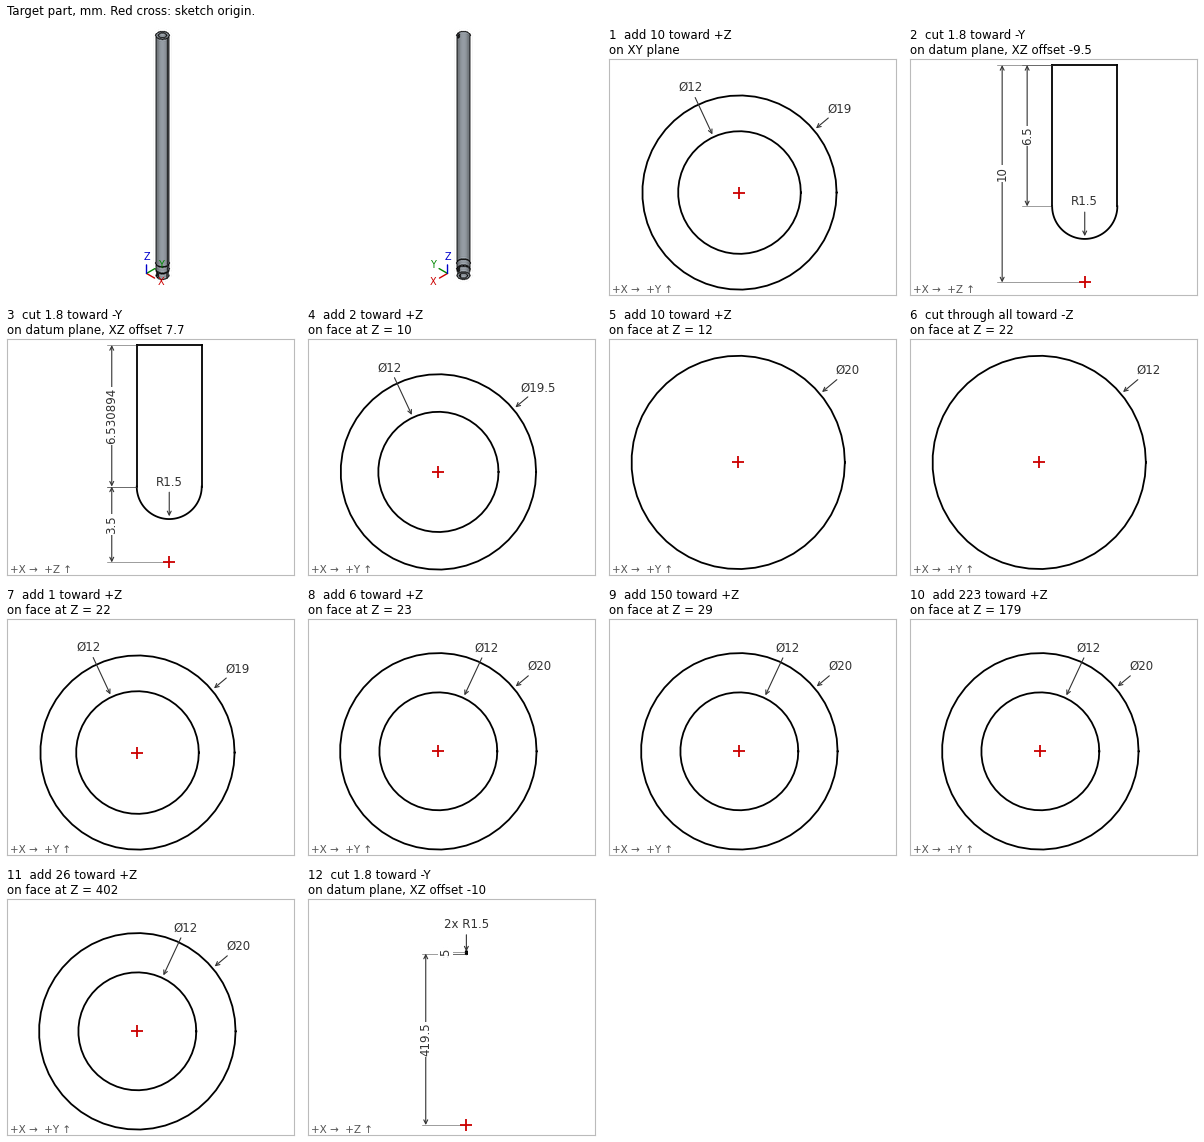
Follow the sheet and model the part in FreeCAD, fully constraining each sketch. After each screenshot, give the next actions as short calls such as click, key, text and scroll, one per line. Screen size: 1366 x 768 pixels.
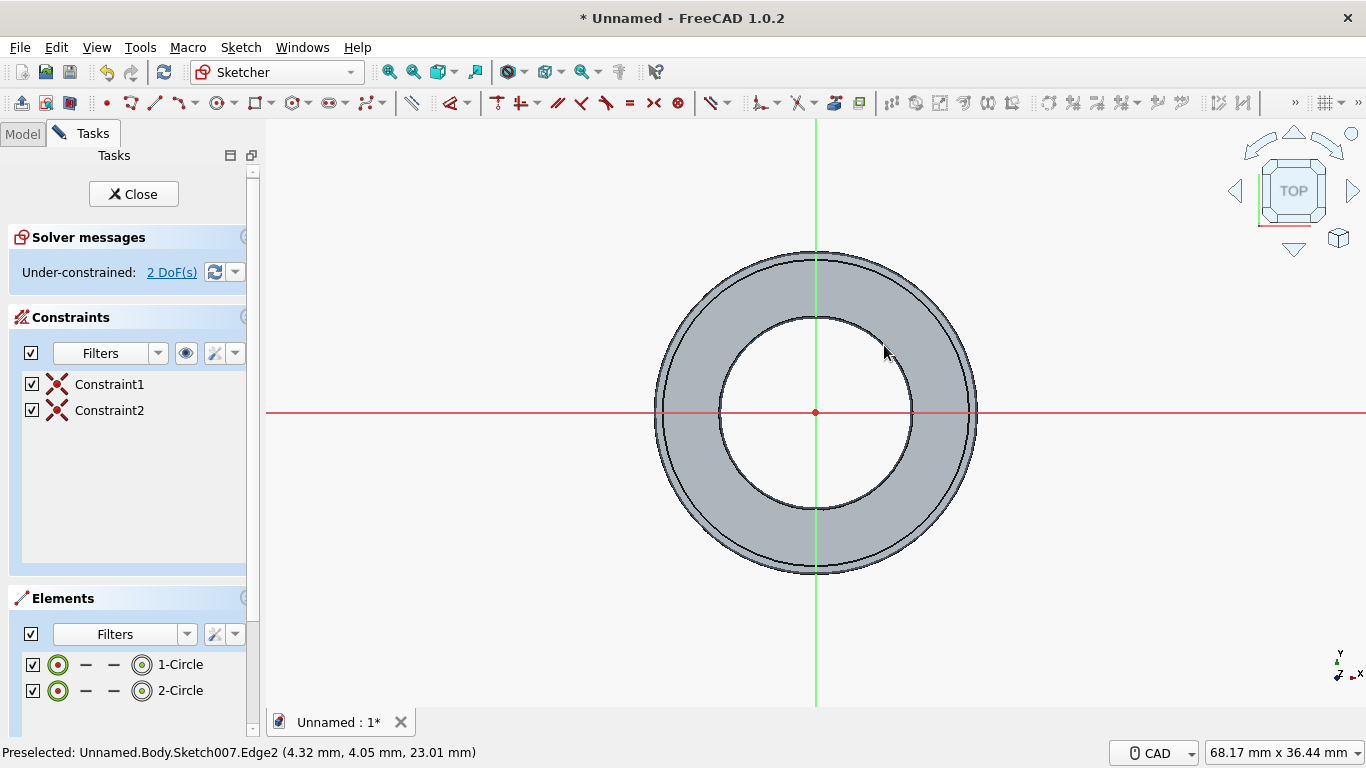
click(450, 104)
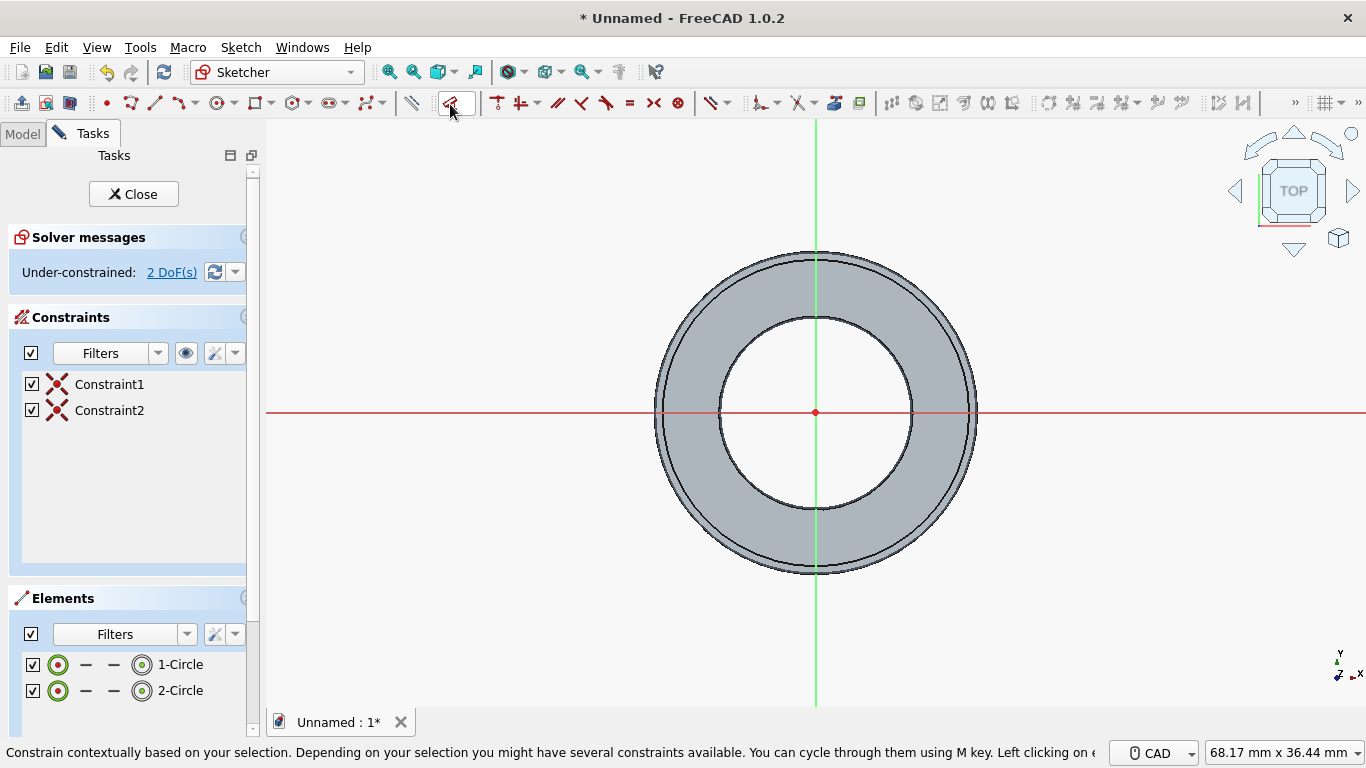
click(929, 299)
click(952, 276)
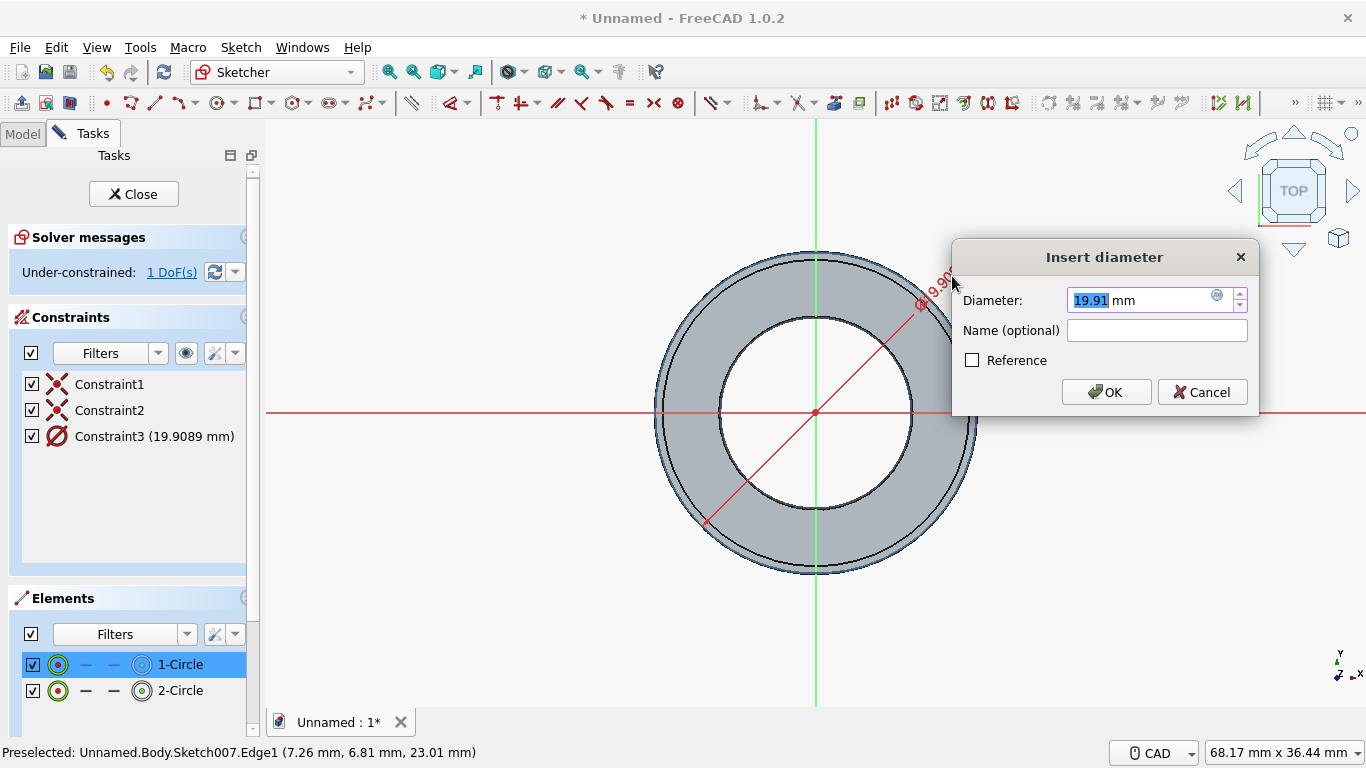
text(20)
key(Return)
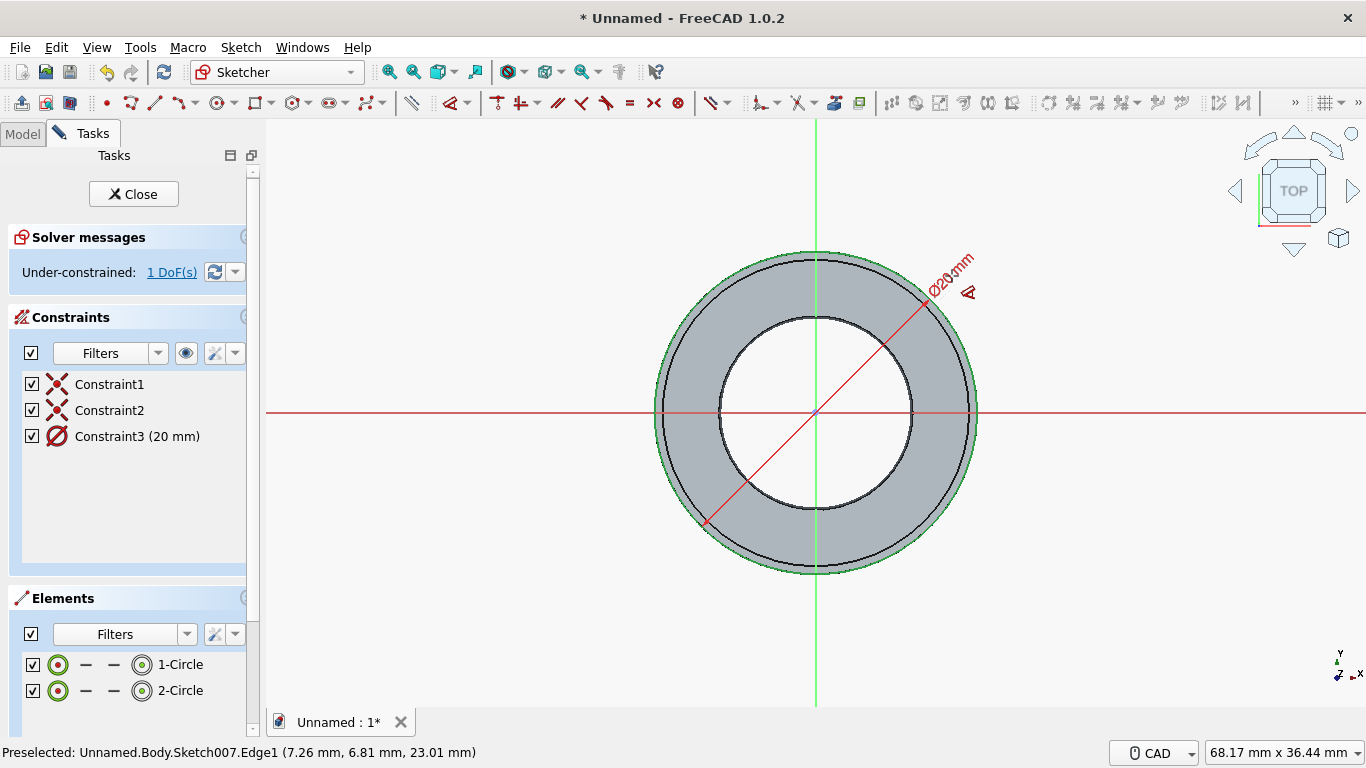
click(883, 345)
click(905, 322)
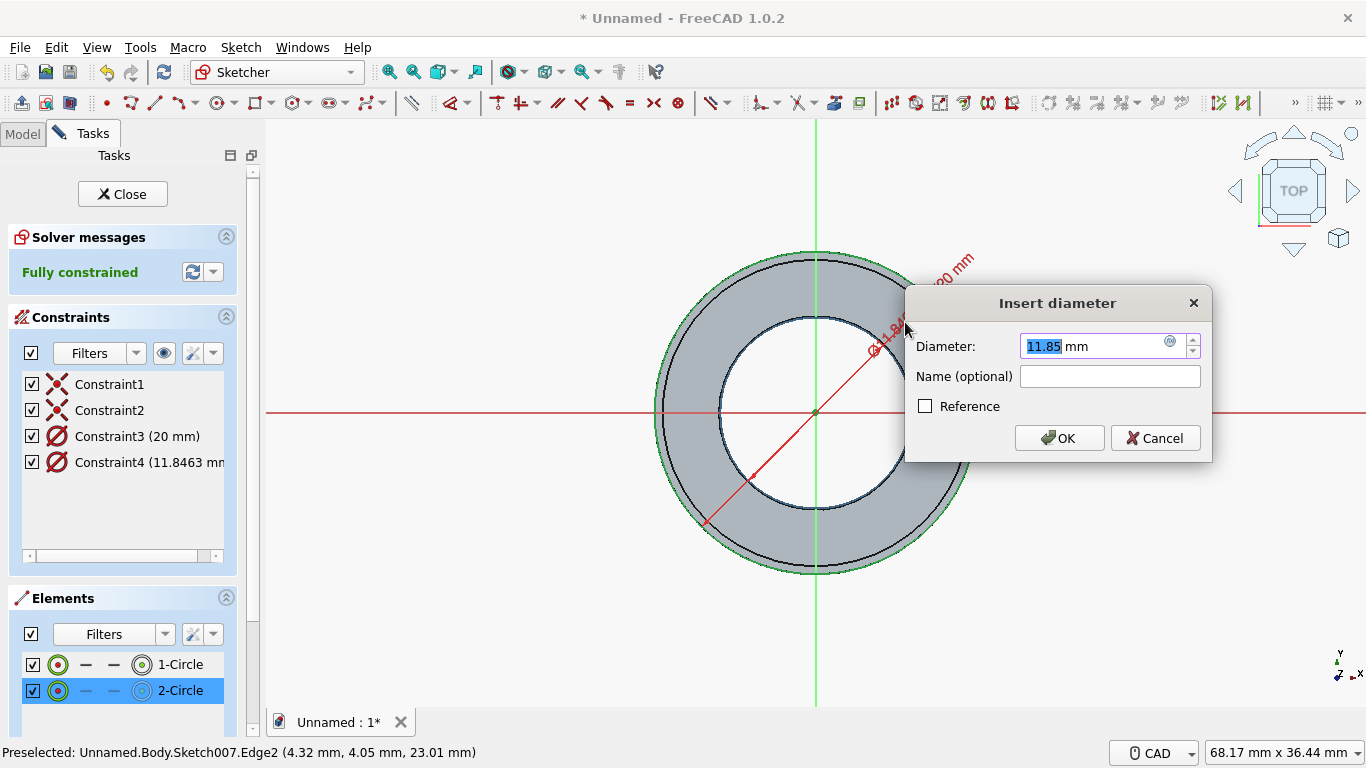
text(12)
key(Return)
key(Escape)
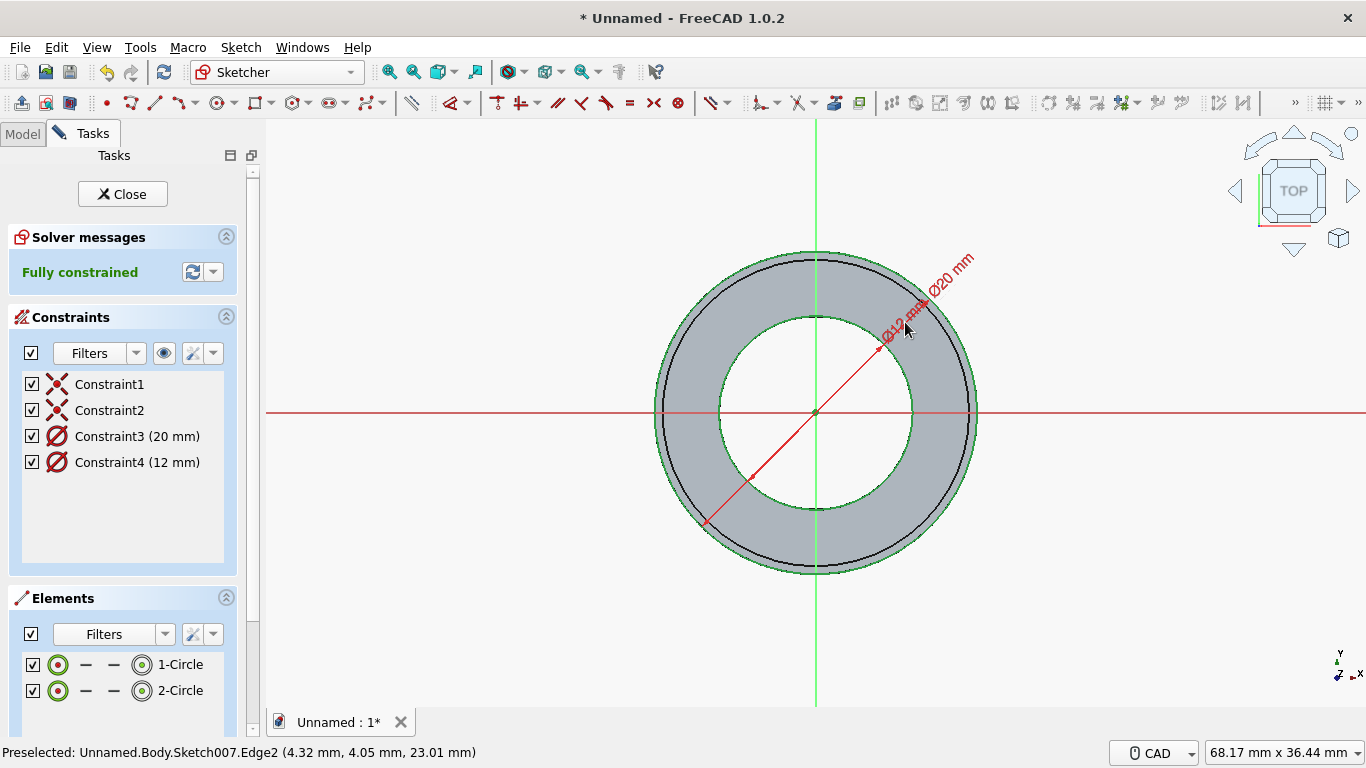
click(123, 194)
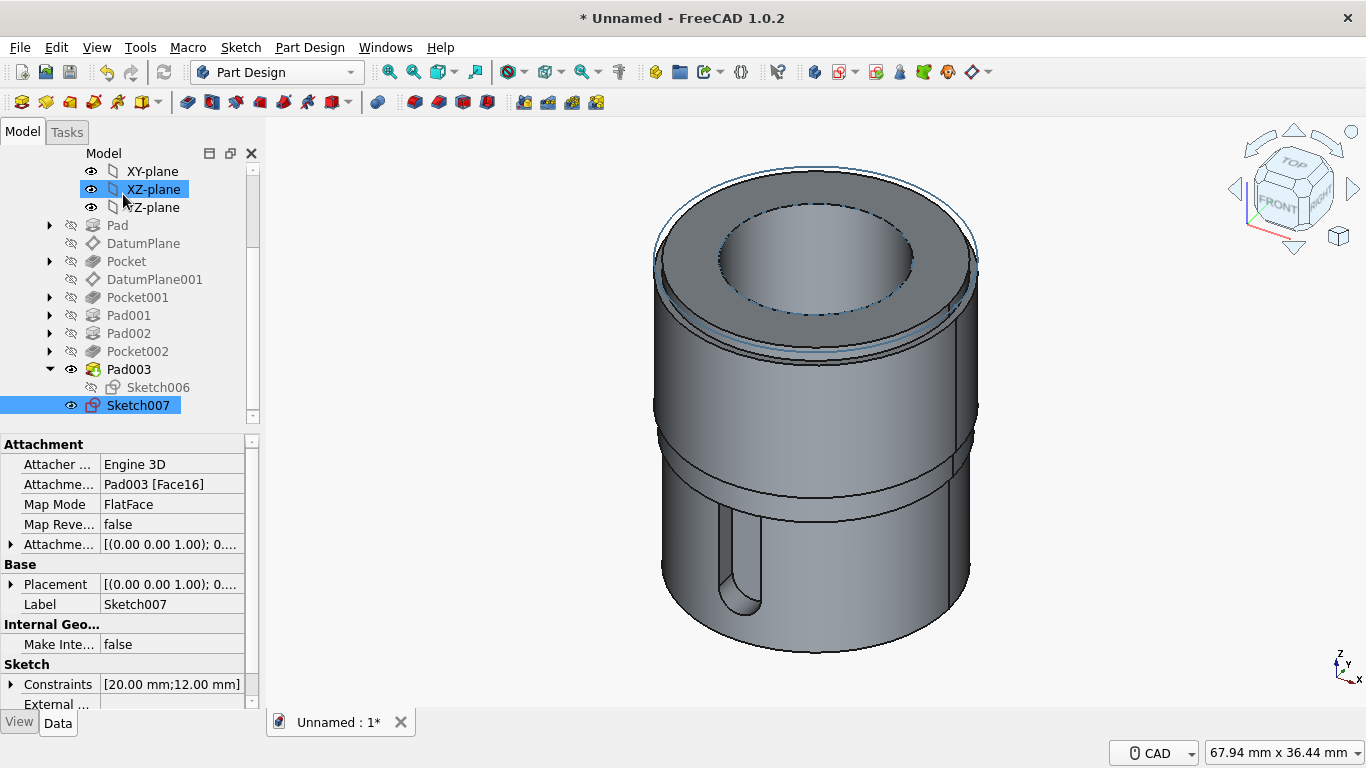
click(22, 102)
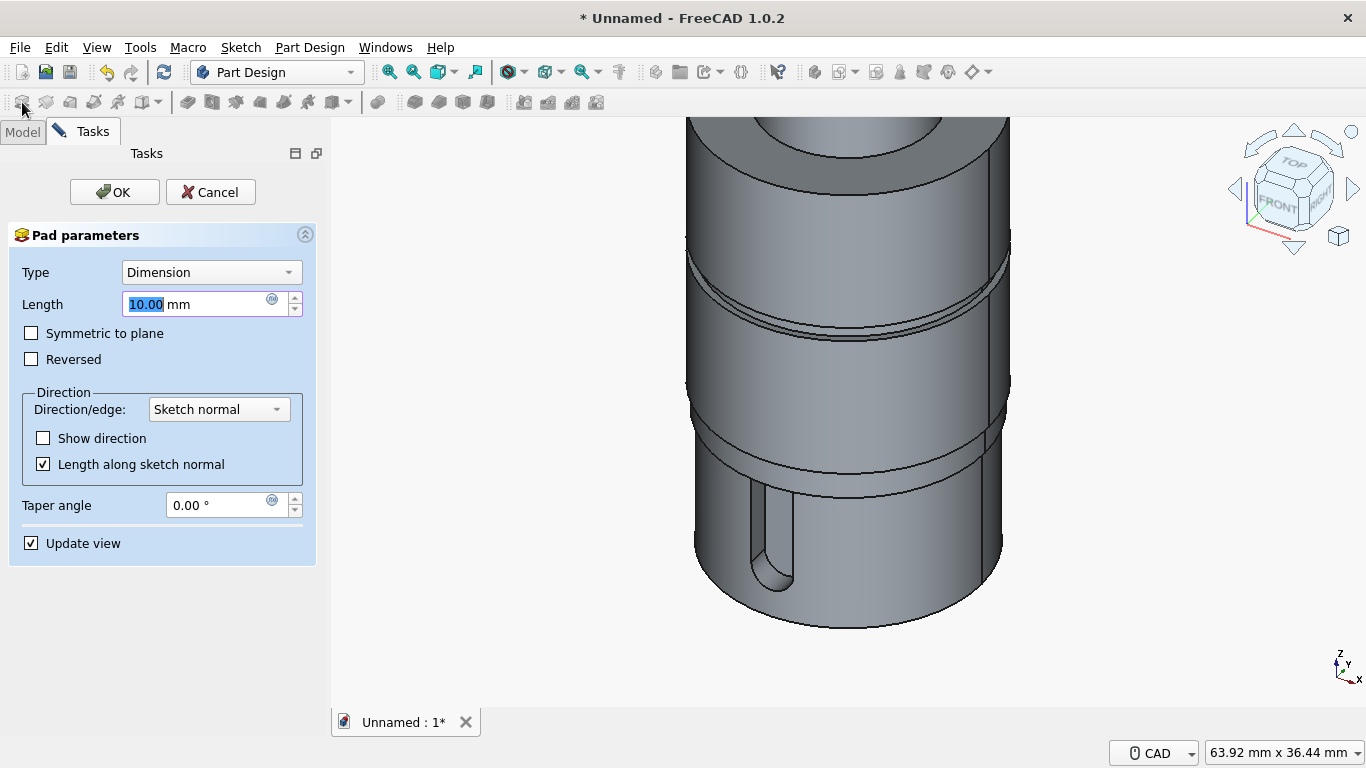
text(6)
key(Tab)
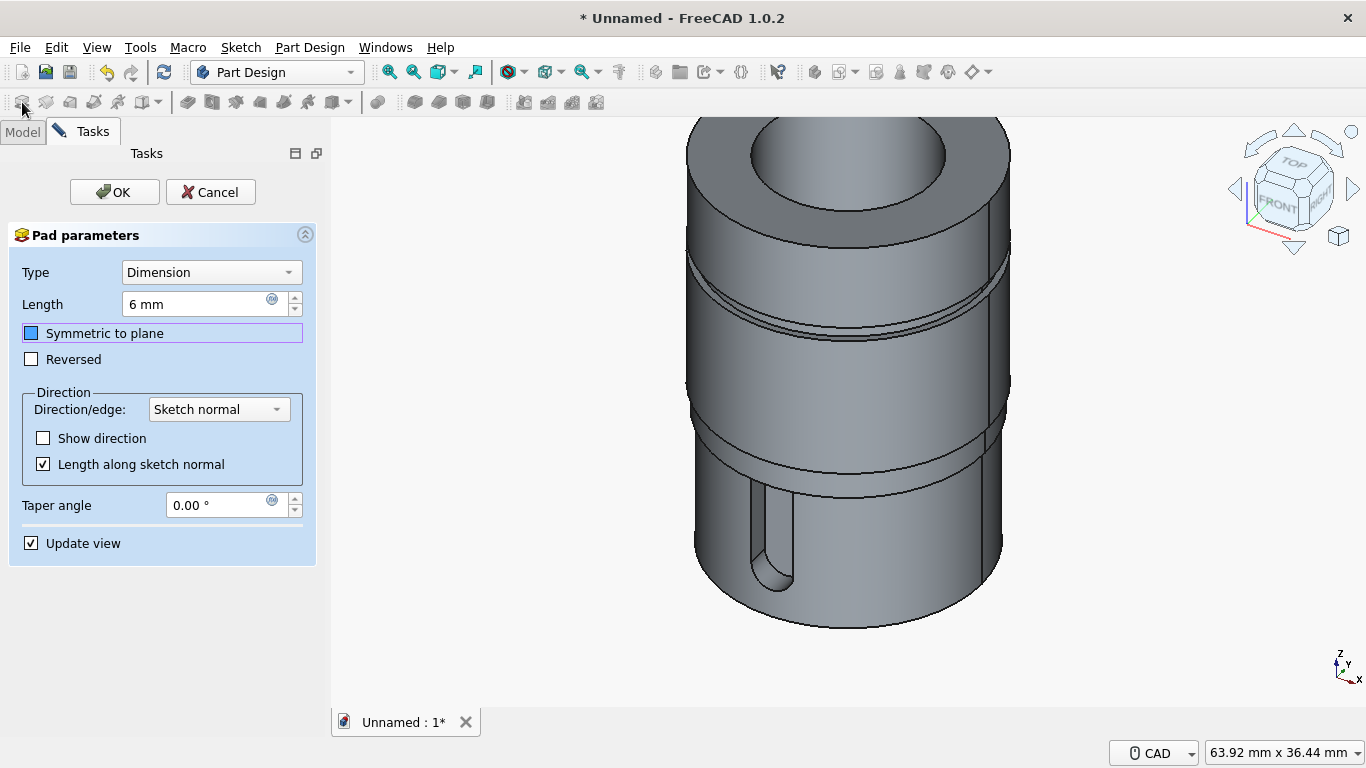
click(115, 192)